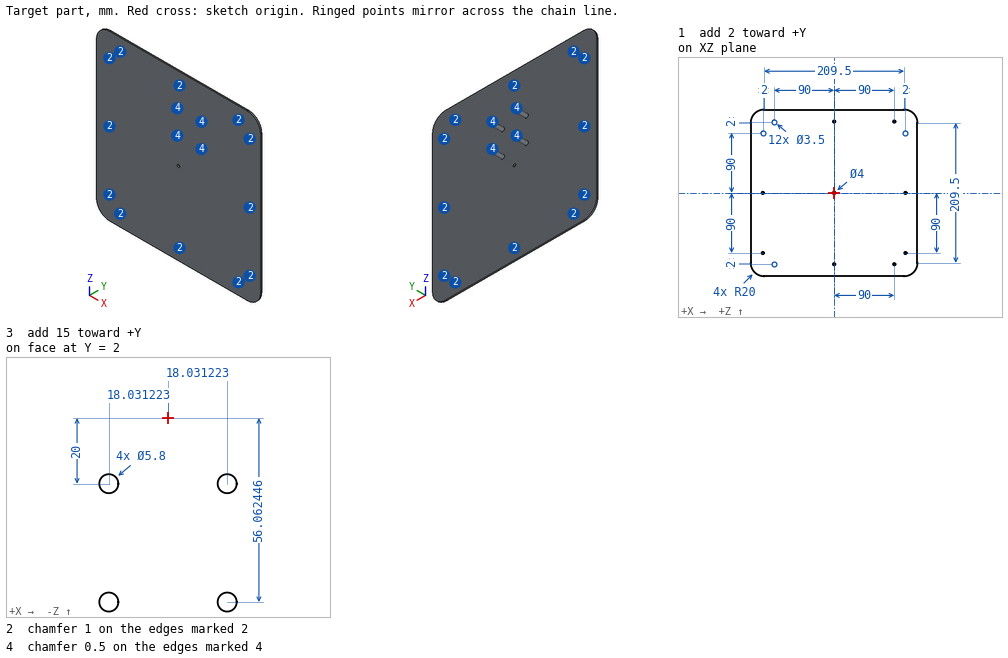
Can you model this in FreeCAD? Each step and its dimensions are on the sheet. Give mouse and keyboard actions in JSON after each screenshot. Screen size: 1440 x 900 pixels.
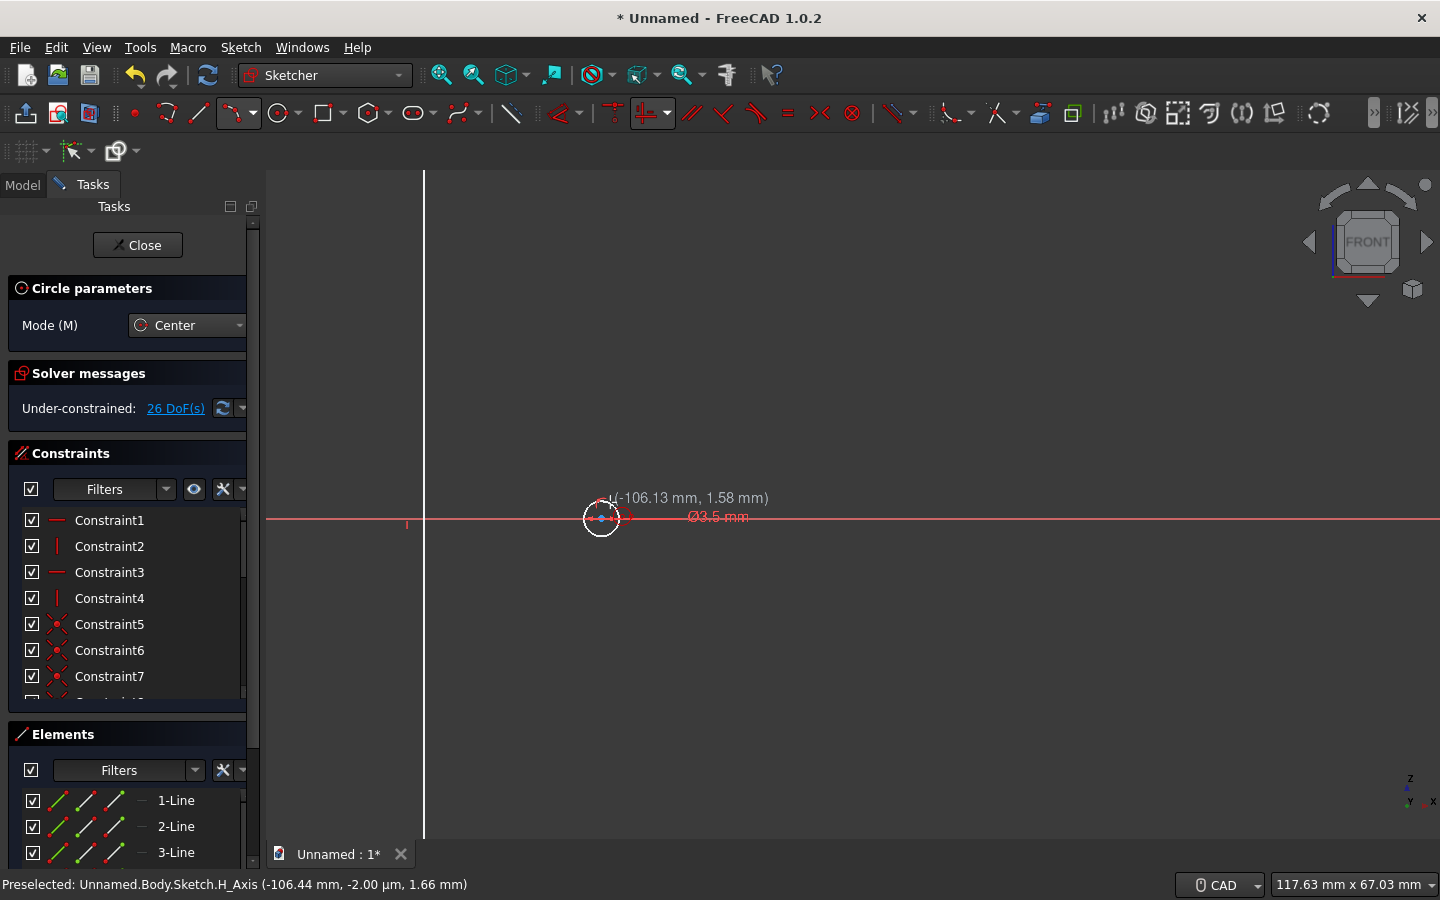
{"action": "scroll", "coordinate": [609, 502], "scroll_direction": "down", "scroll_amount": 9}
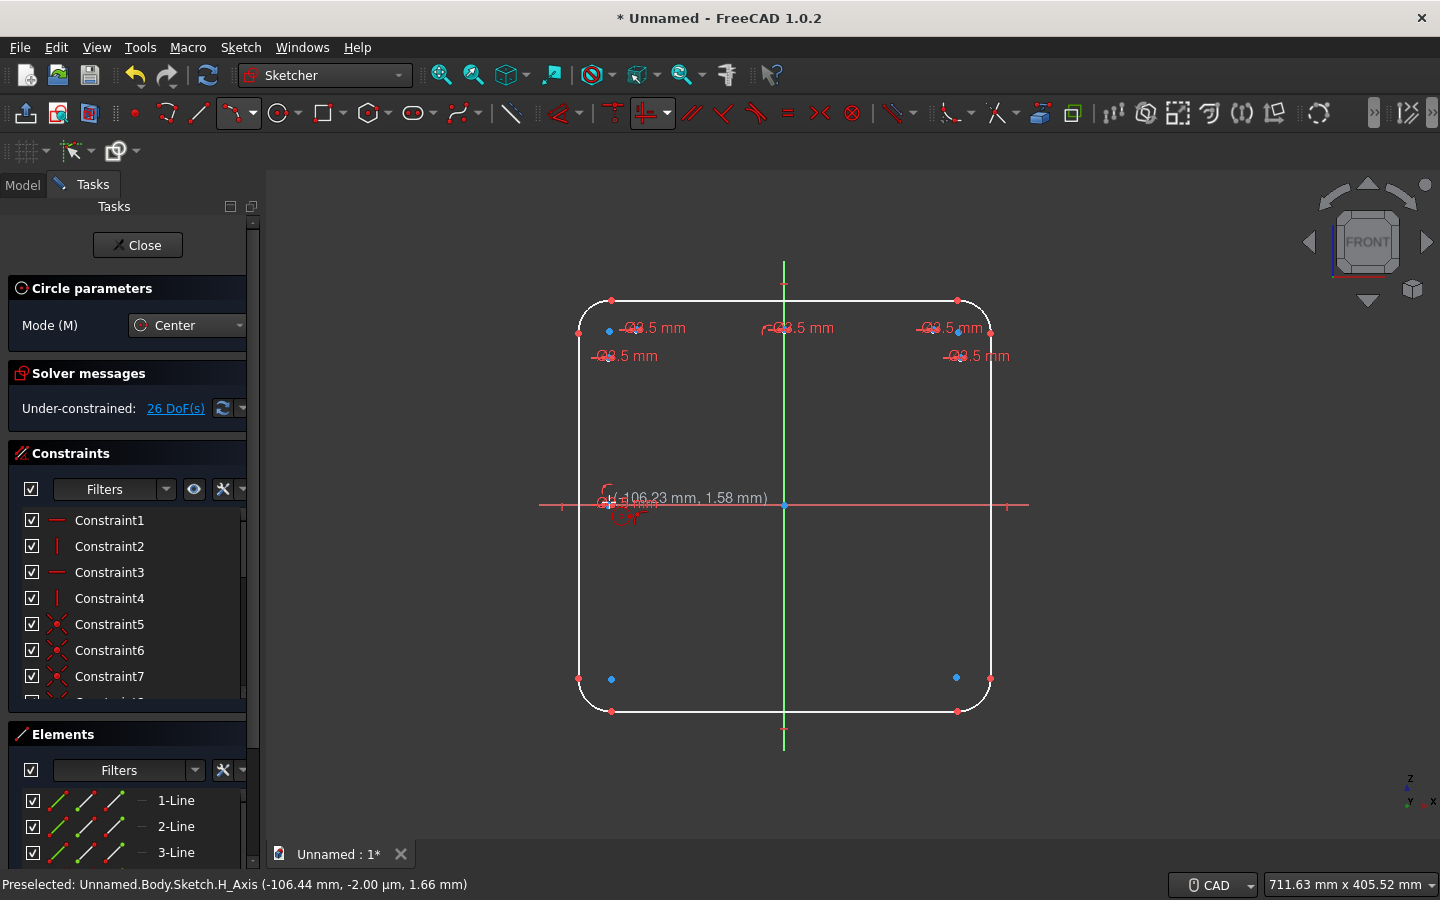
{"action": "scroll", "coordinate": [608, 654], "scroll_direction": "up", "scroll_amount": 11}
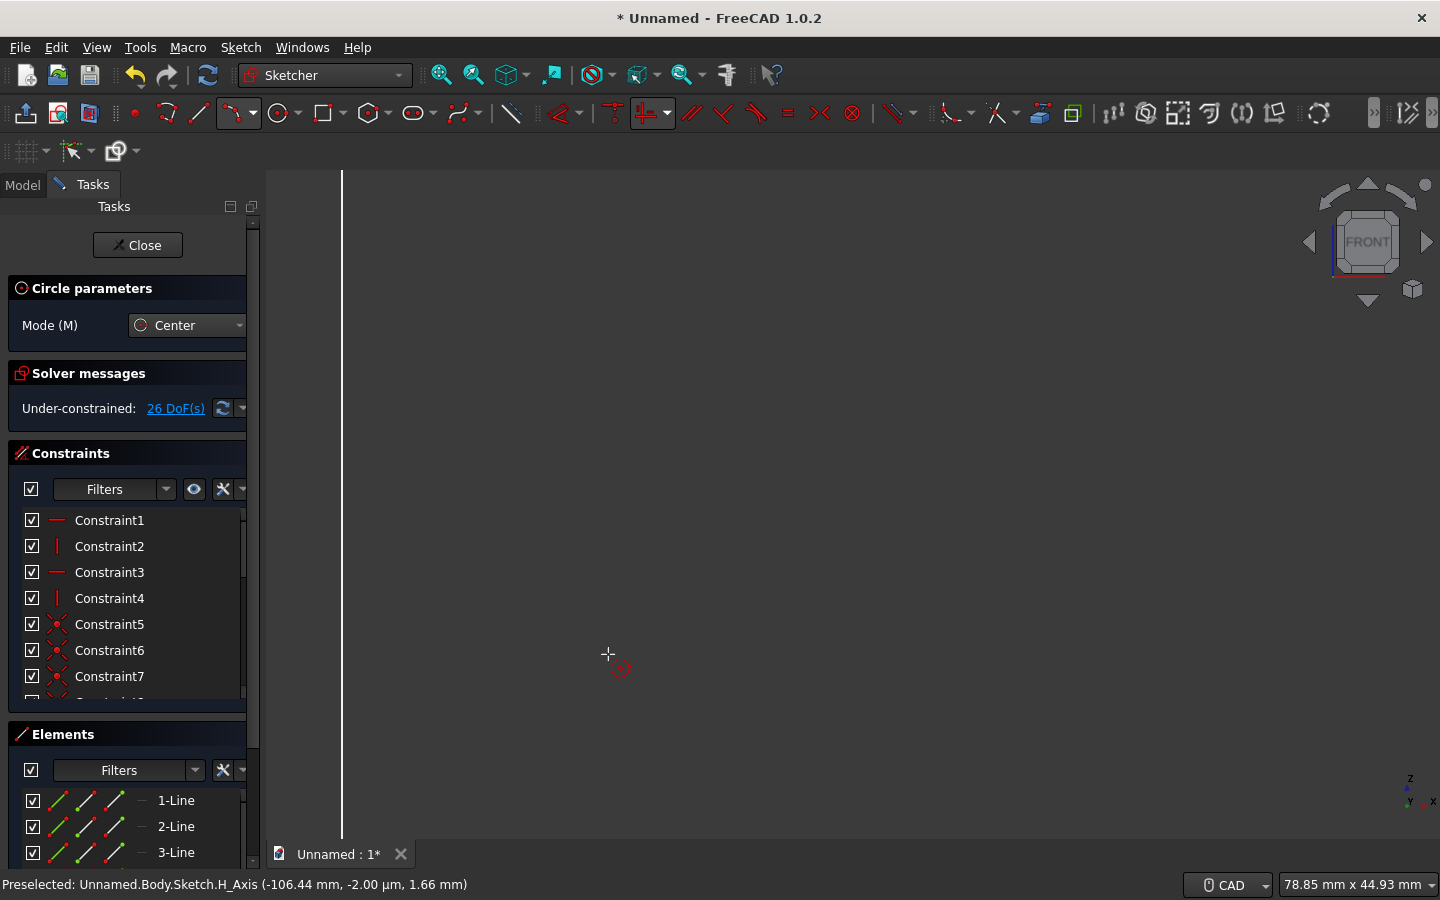
{"action": "scroll", "coordinate": [608, 654], "scroll_direction": "down", "scroll_amount": 11}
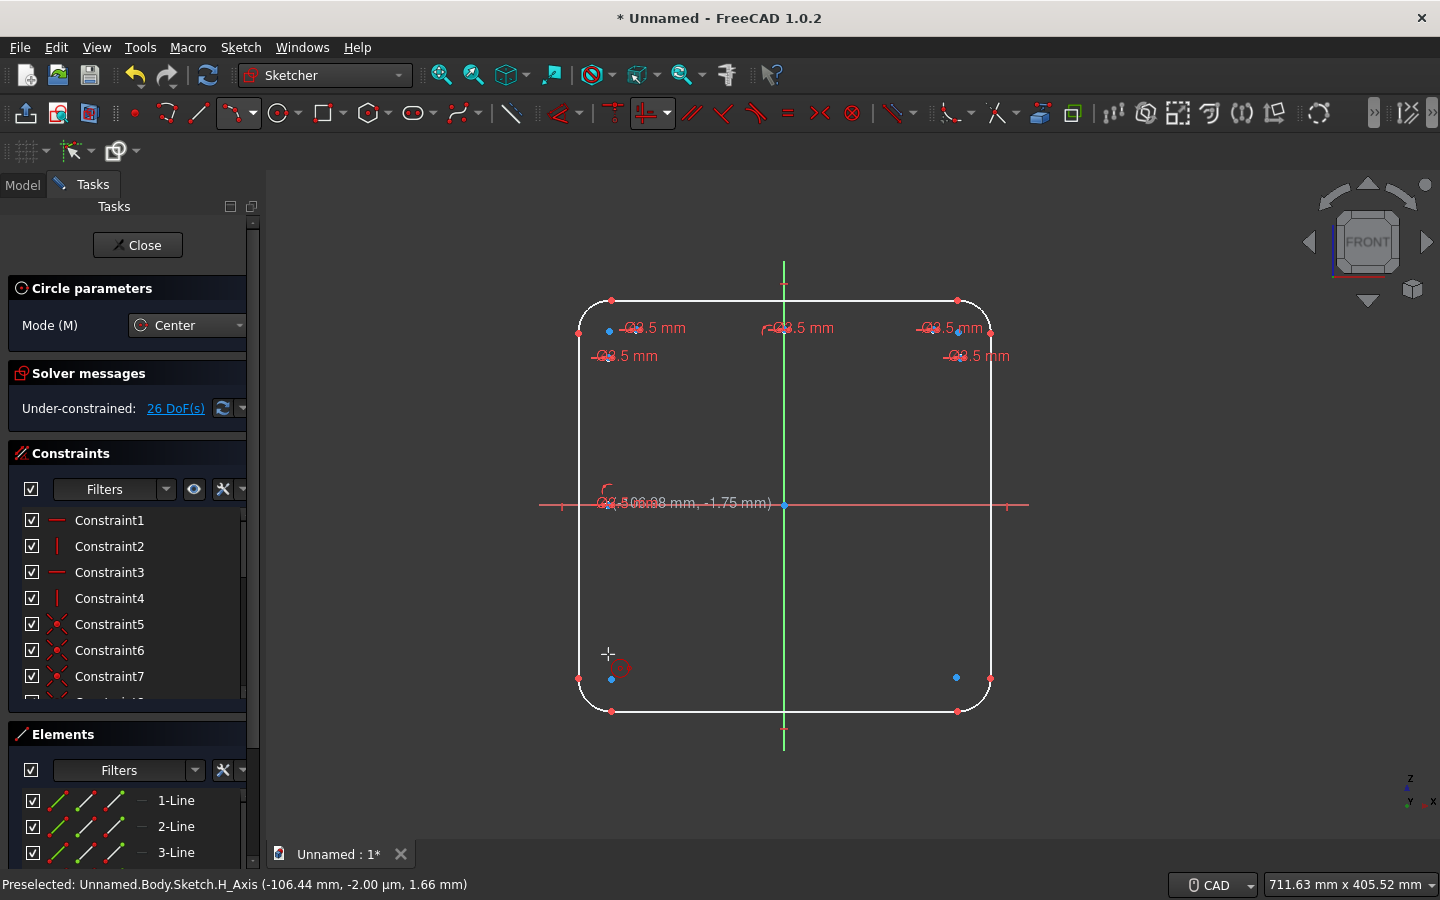
{"action": "left_click", "coordinate": [608, 654]}
{"action": "mouse_move", "coordinate": [610, 652]}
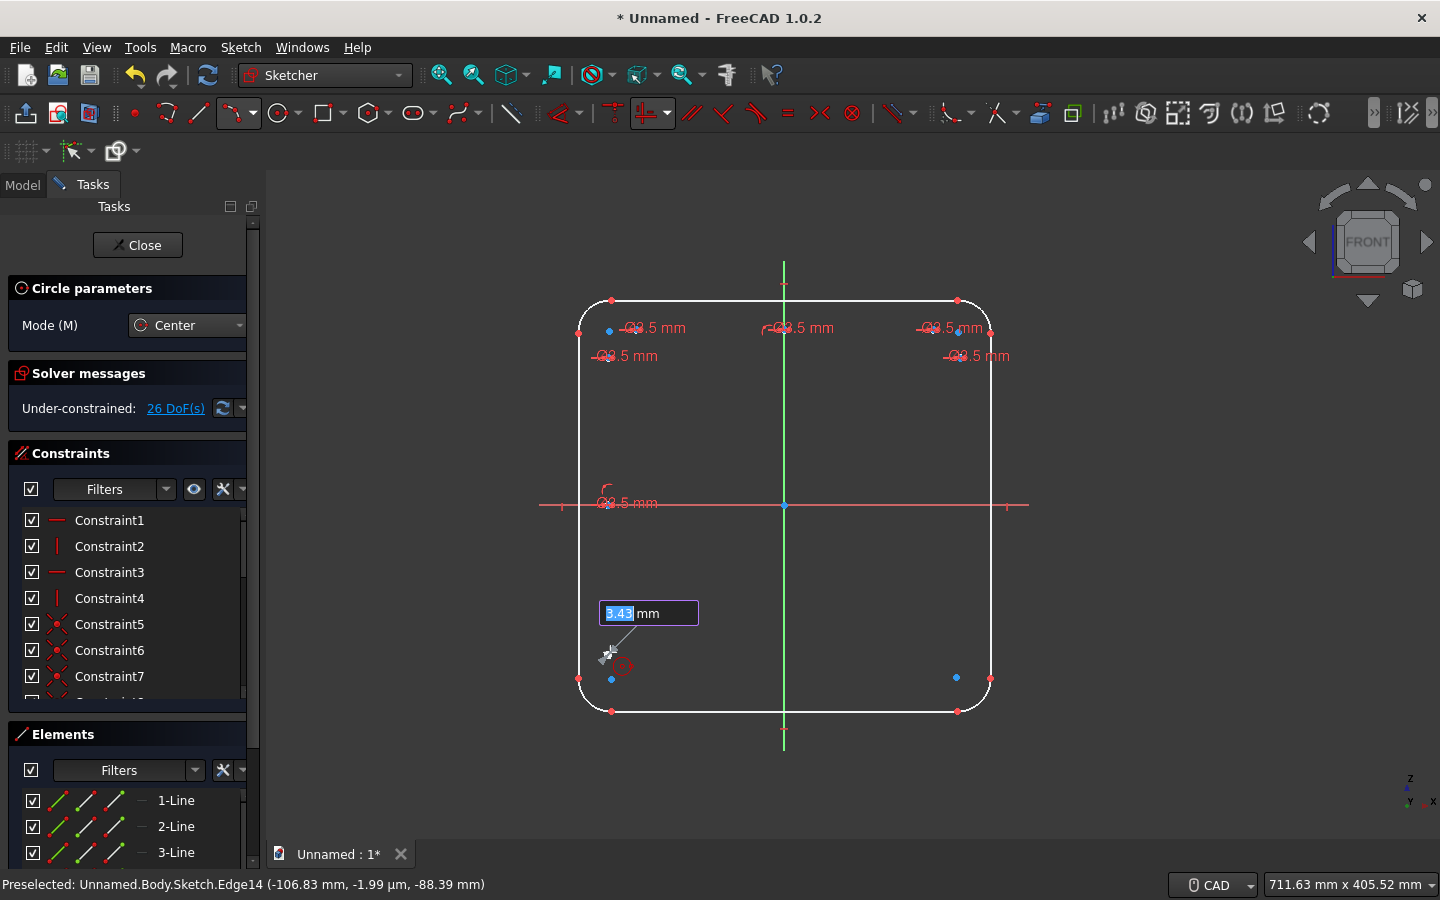
{"action": "type", "text": "3.5"}
{"action": "key", "text": "Return"}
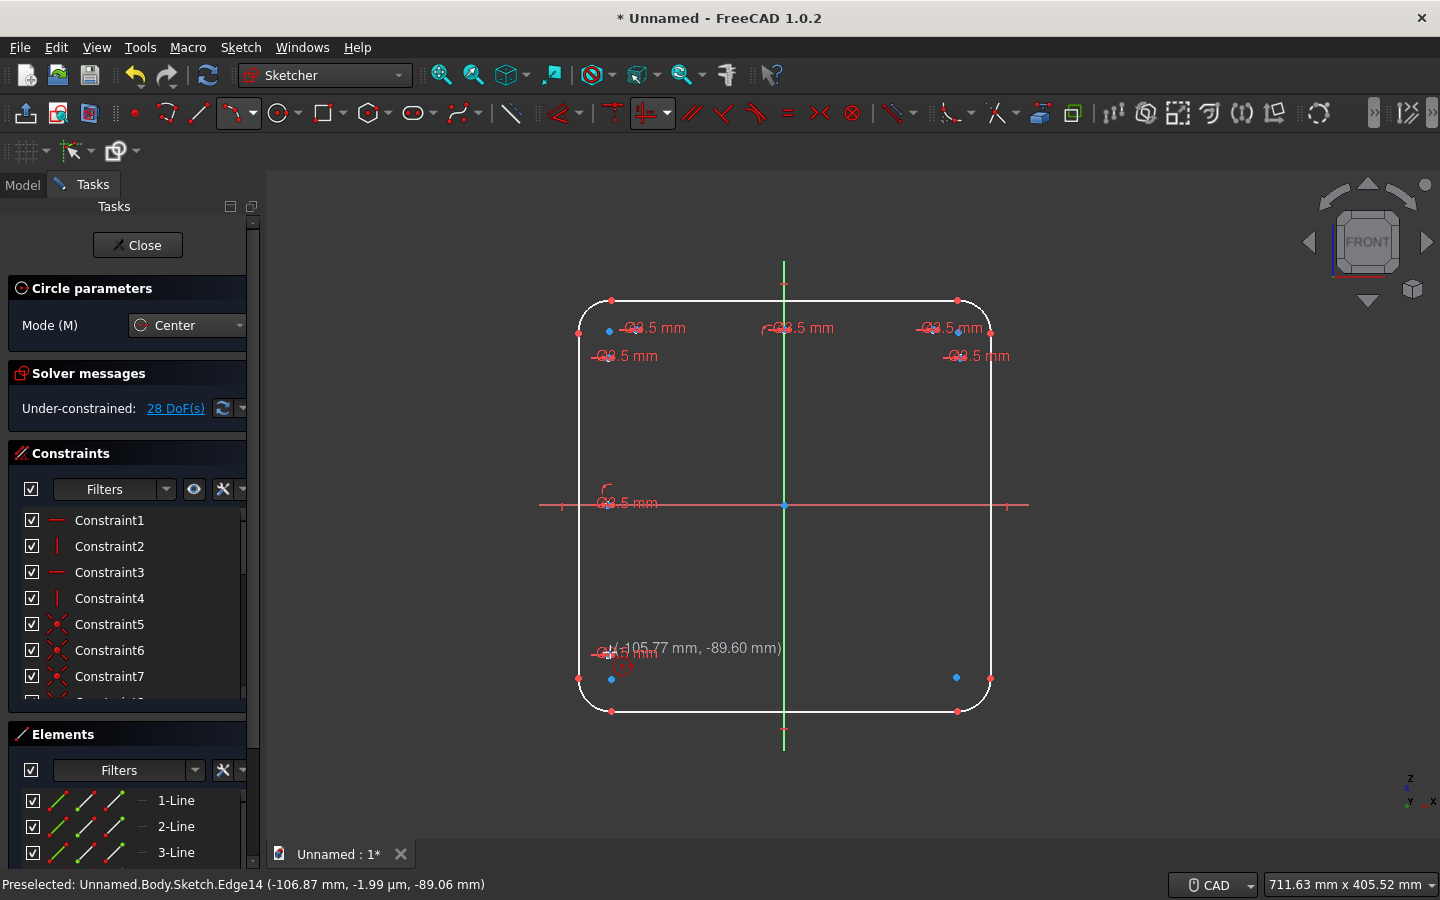
{"action": "scroll", "coordinate": [636, 681], "scroll_direction": "up", "scroll_amount": 11}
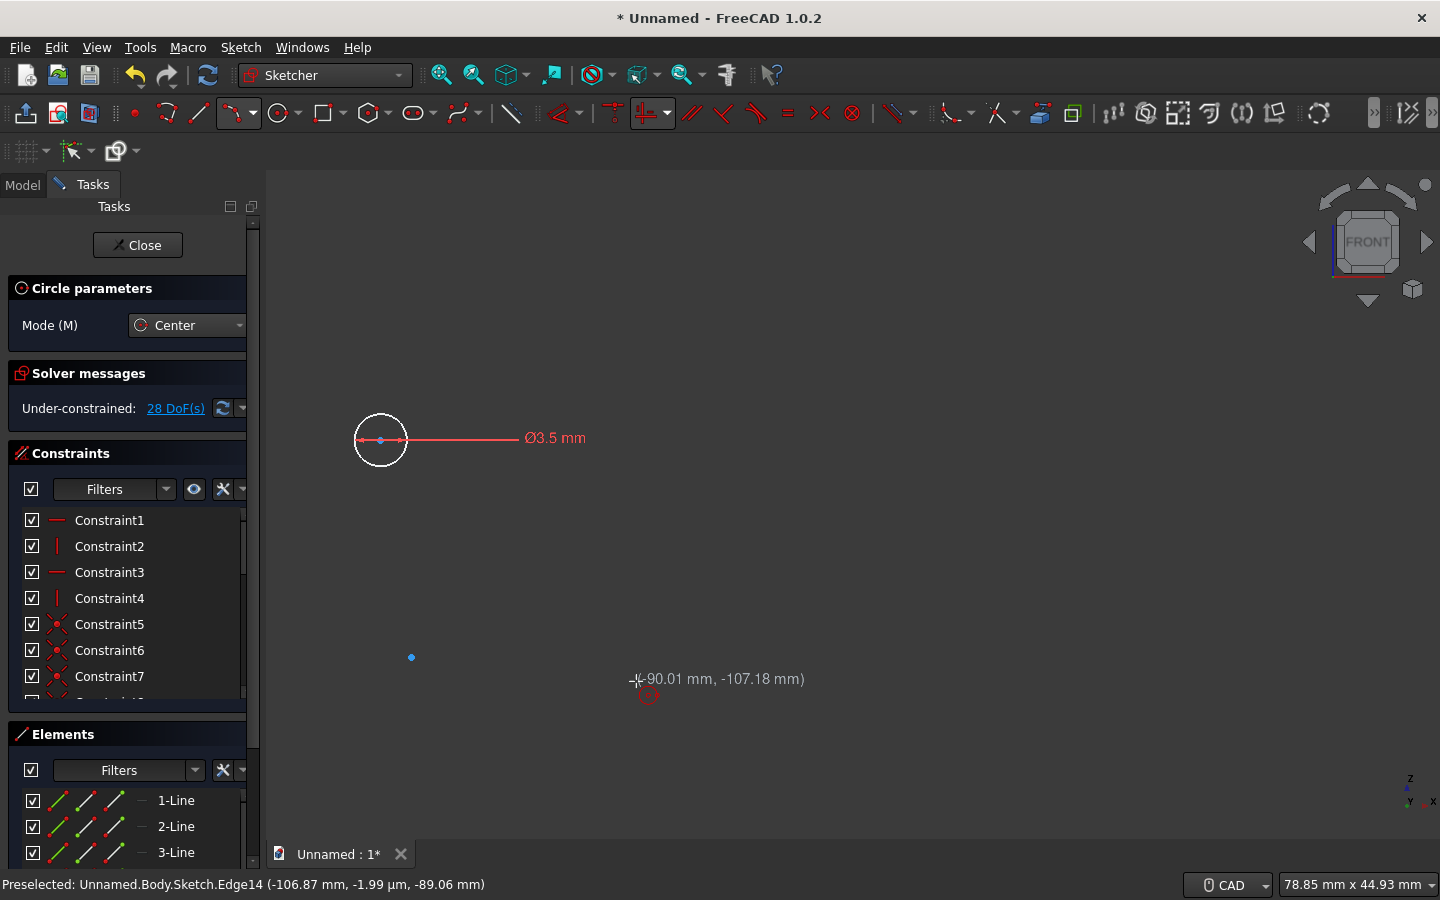
{"action": "scroll", "coordinate": [636, 681], "scroll_direction": "down", "scroll_amount": 11}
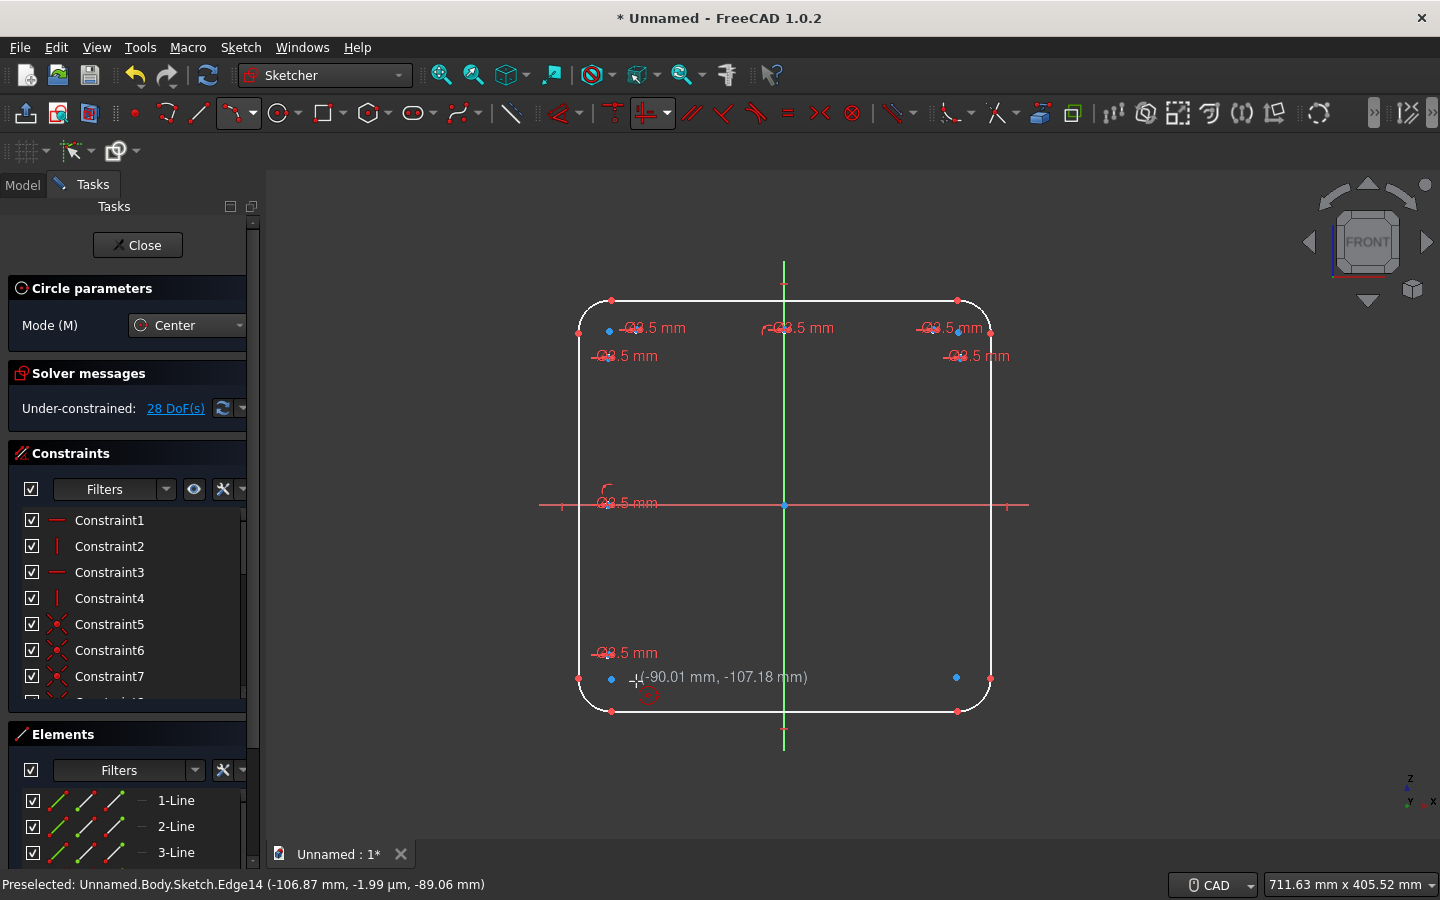
{"action": "left_click", "coordinate": [636, 681]}
{"action": "mouse_move", "coordinate": [638, 679]}